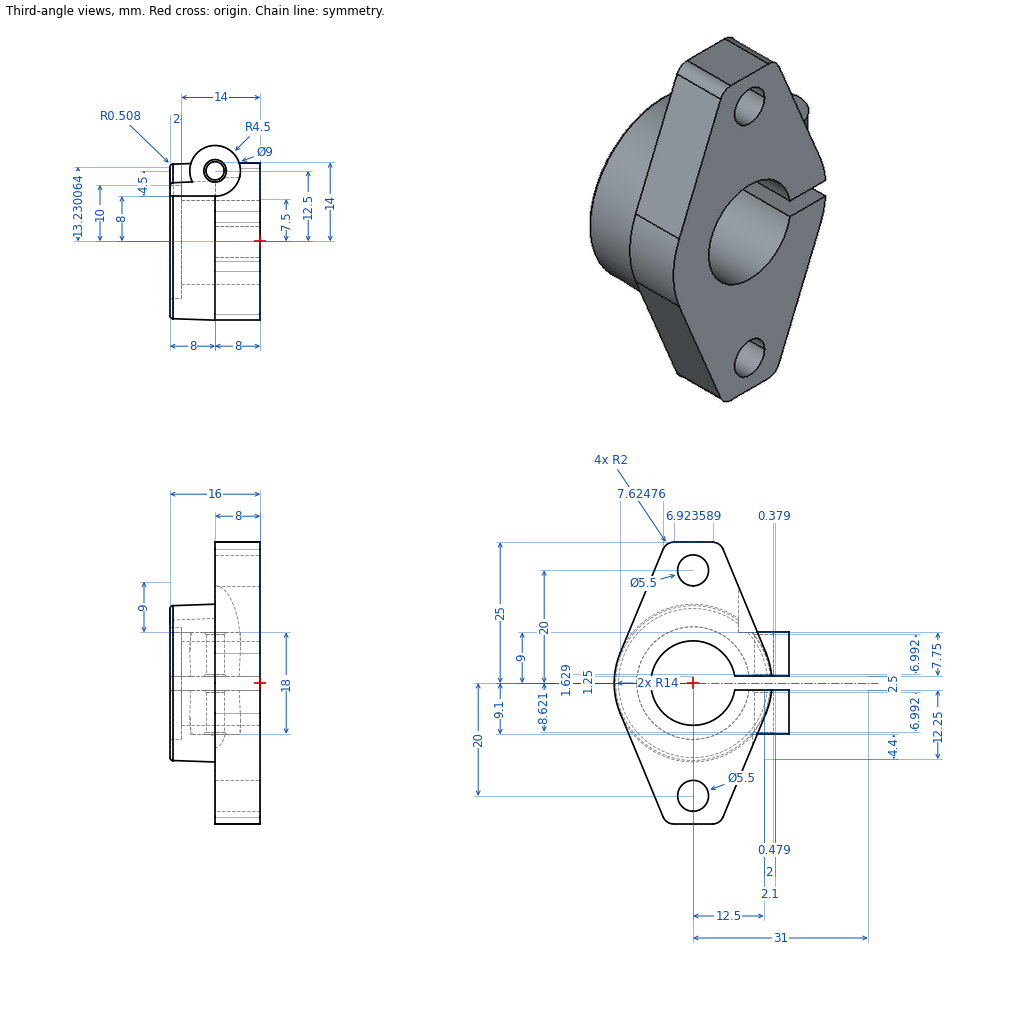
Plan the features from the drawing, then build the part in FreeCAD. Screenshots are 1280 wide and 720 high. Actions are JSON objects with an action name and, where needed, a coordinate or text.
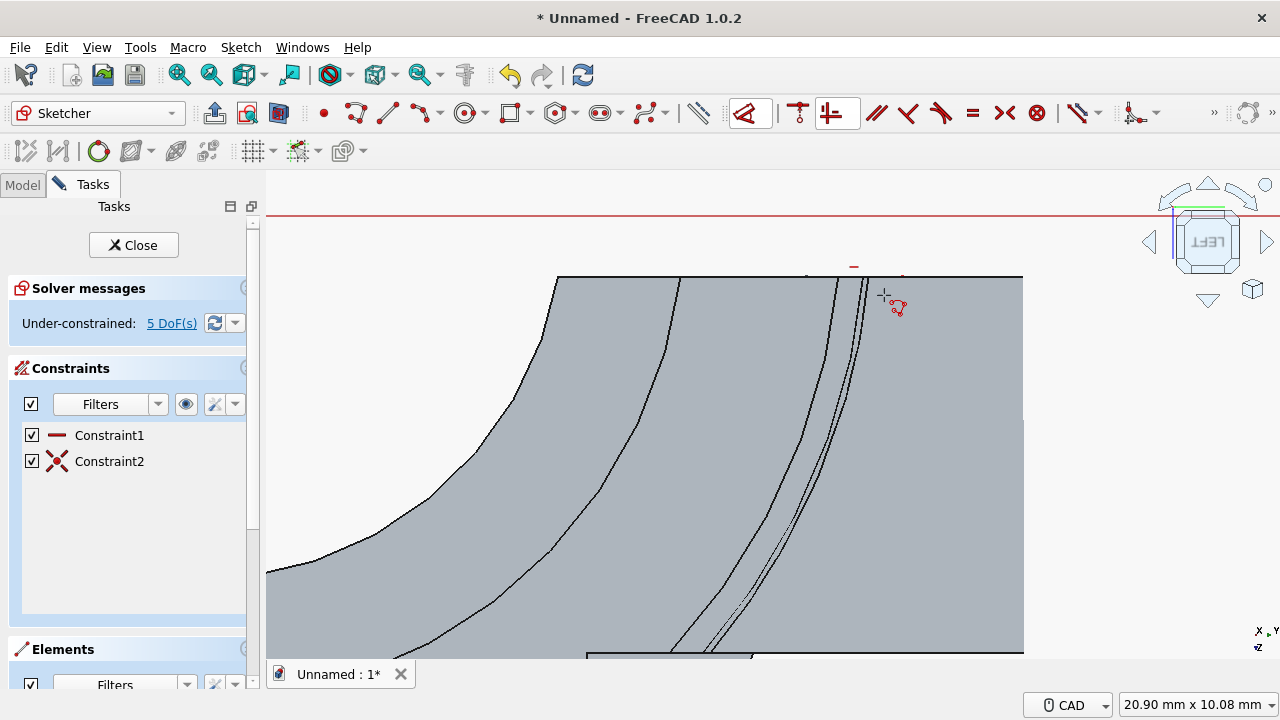
{"action": "scroll", "coordinate": [891, 299], "scroll_direction": "down", "scroll_amount": 3}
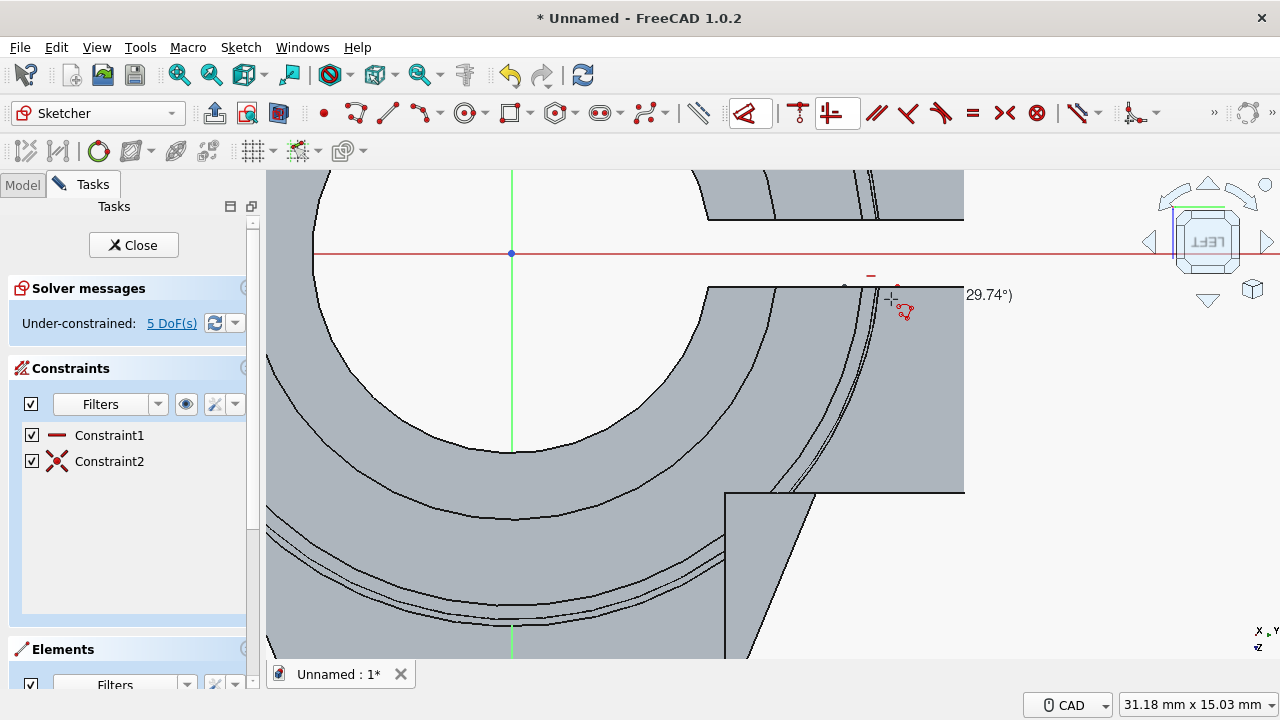
{"action": "left_click", "coordinate": [887, 483]}
{"action": "left_click", "coordinate": [898, 493]}
{"action": "left_click", "coordinate": [845, 493]}
{"action": "left_click", "coordinate": [845, 288]}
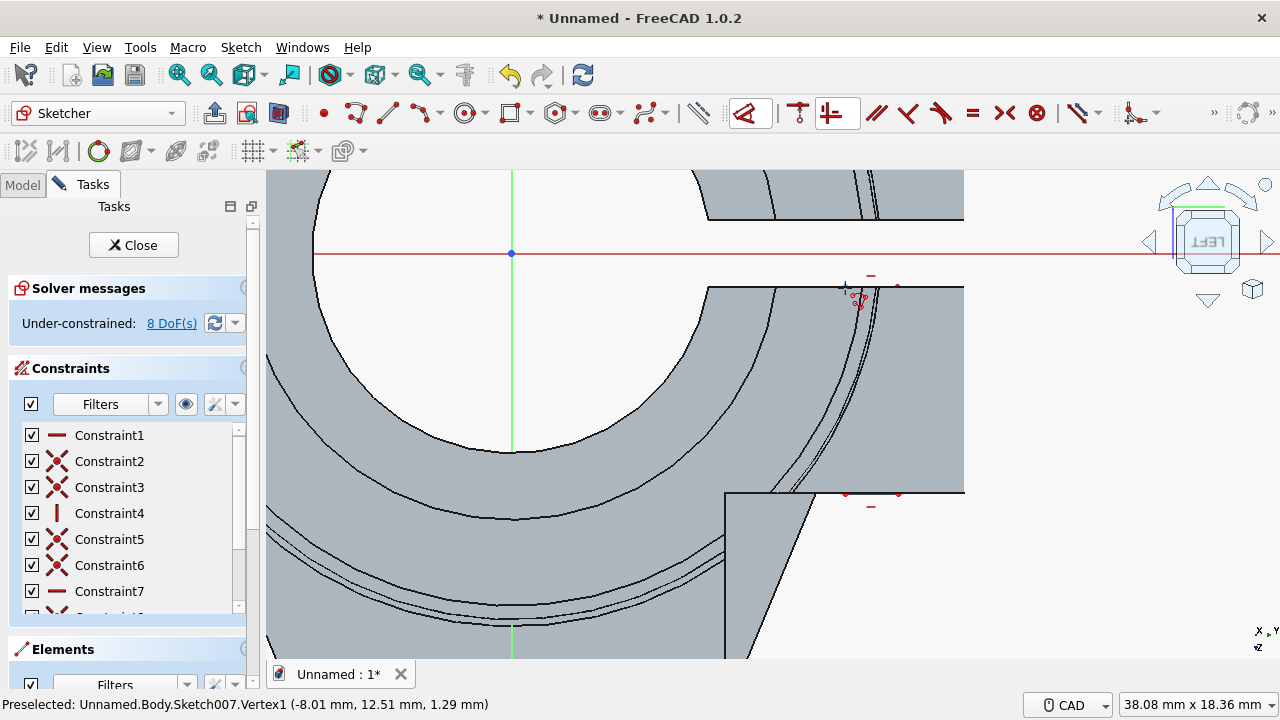
{"action": "left_click", "coordinate": [388, 114]}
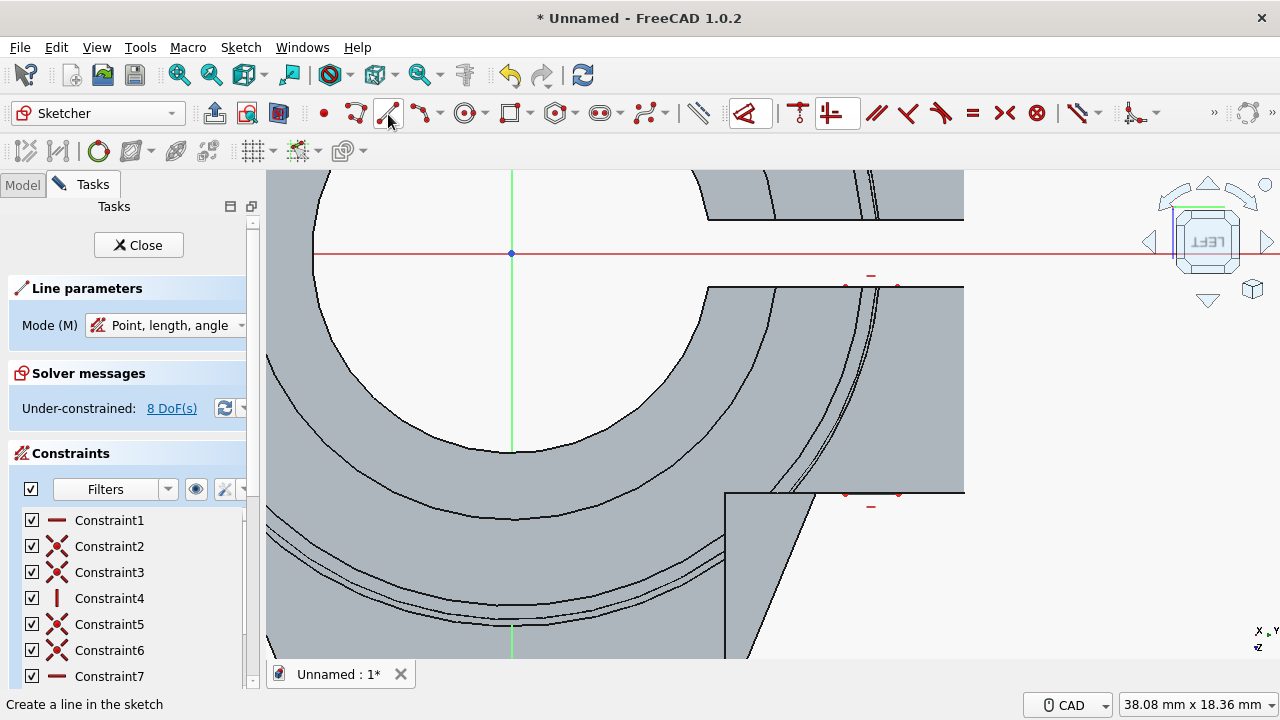
{"action": "left_click", "coordinate": [845, 514]}
{"action": "left_click", "coordinate": [845, 576]}
{"action": "key", "text": "Escape"}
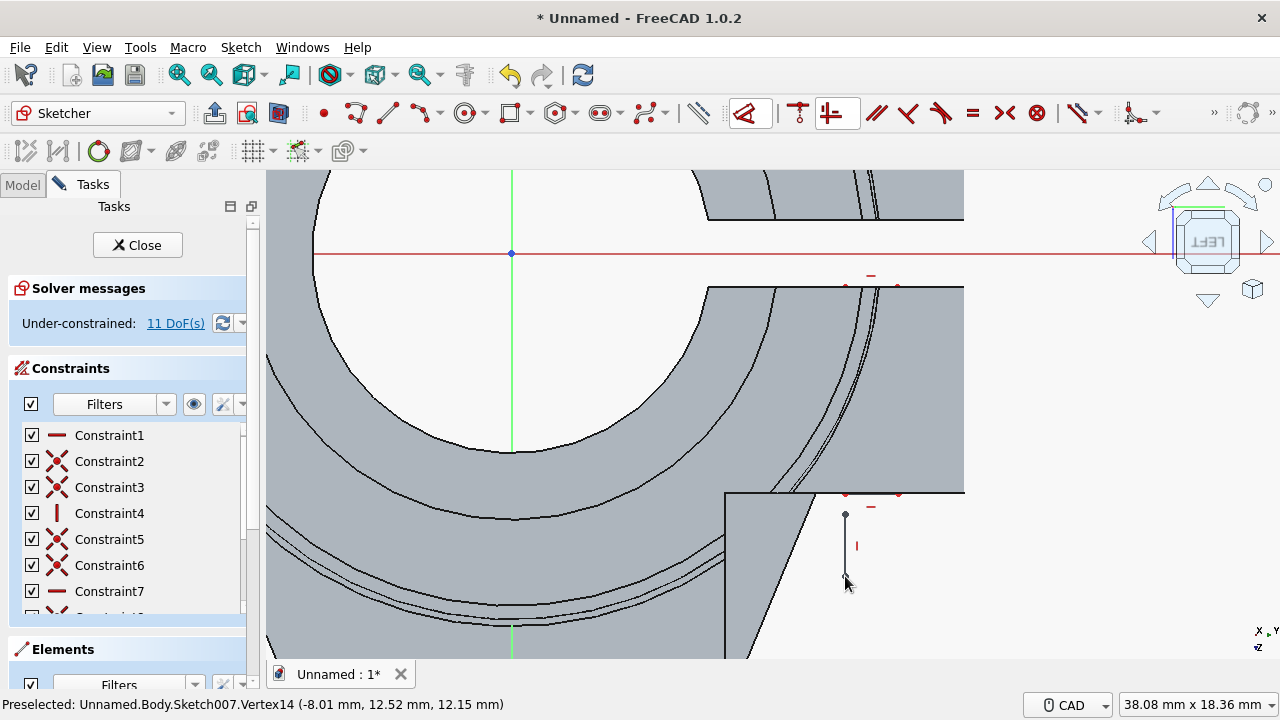
{"action": "left_click", "coordinate": [845, 534]}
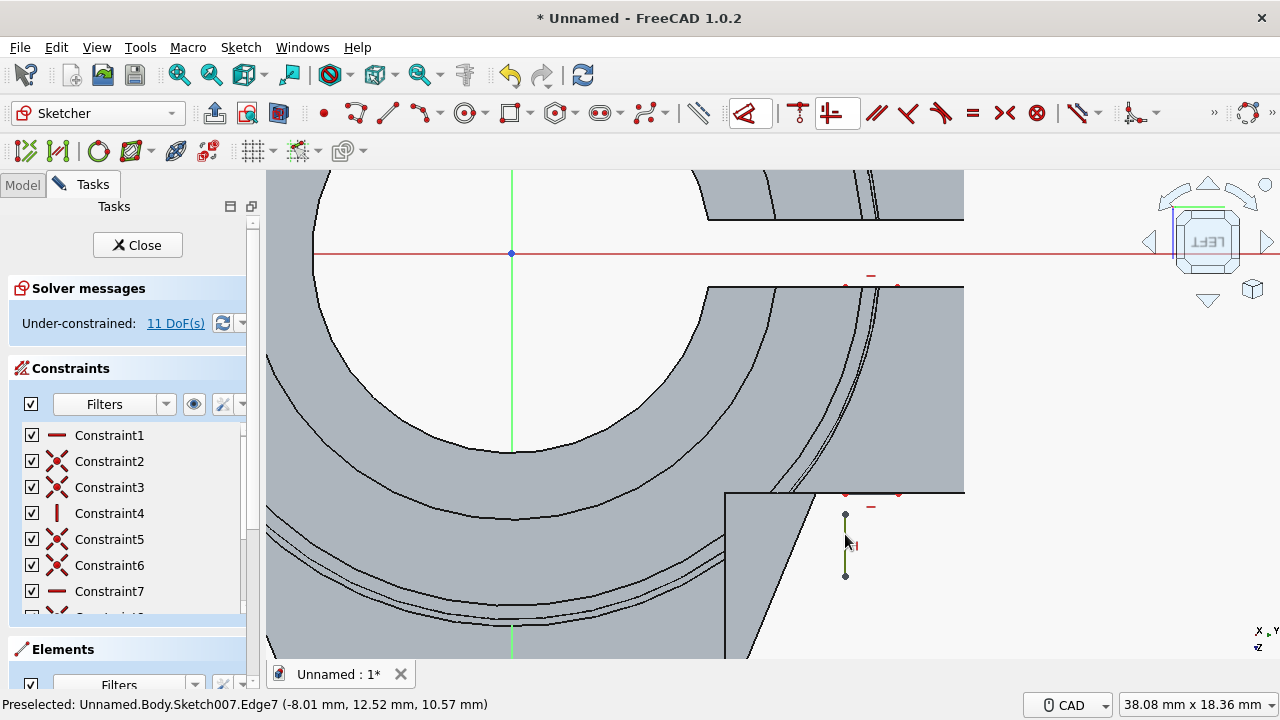
{"action": "left_click", "coordinate": [700, 114]}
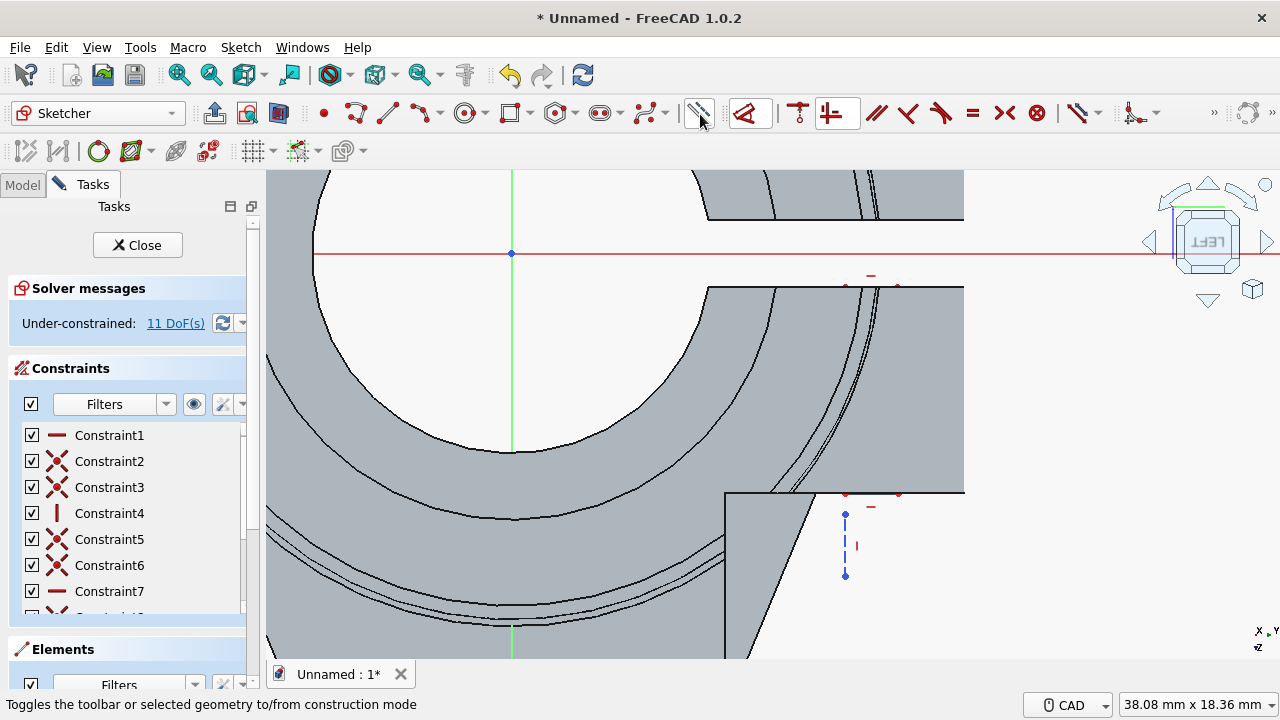
{"action": "left_click", "coordinate": [861, 288]}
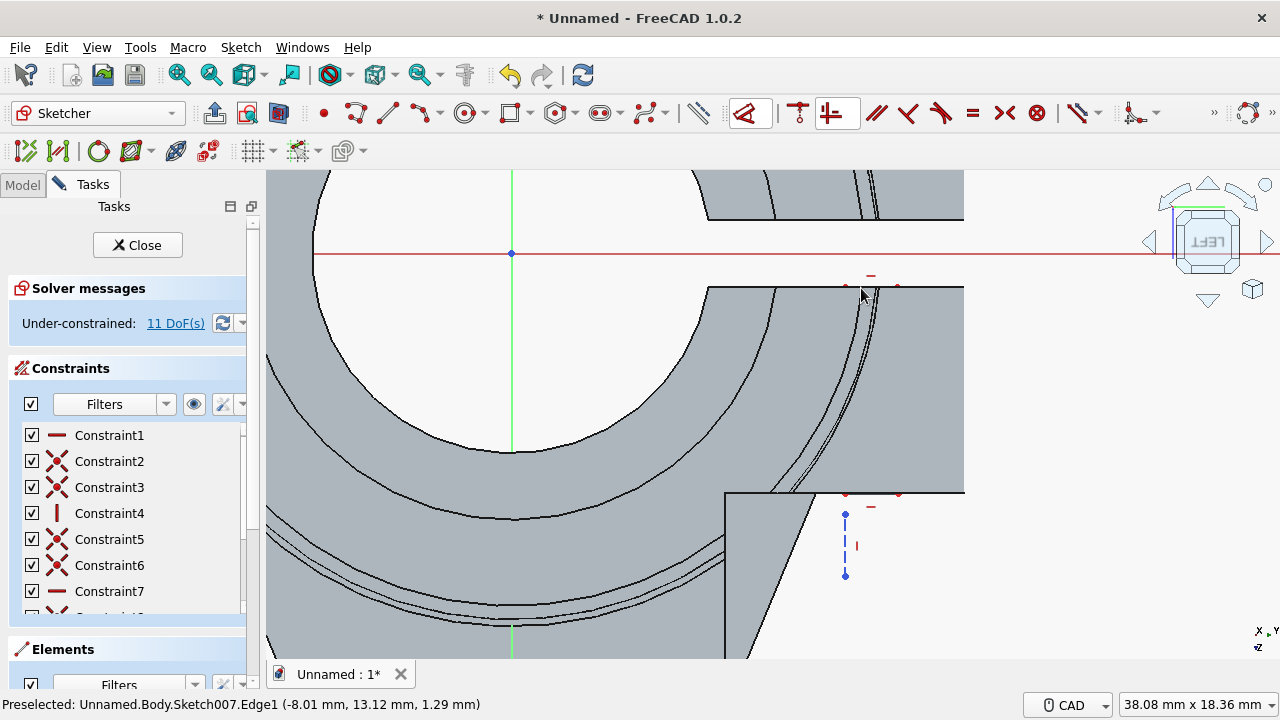
{"action": "left_click", "coordinate": [766, 114]}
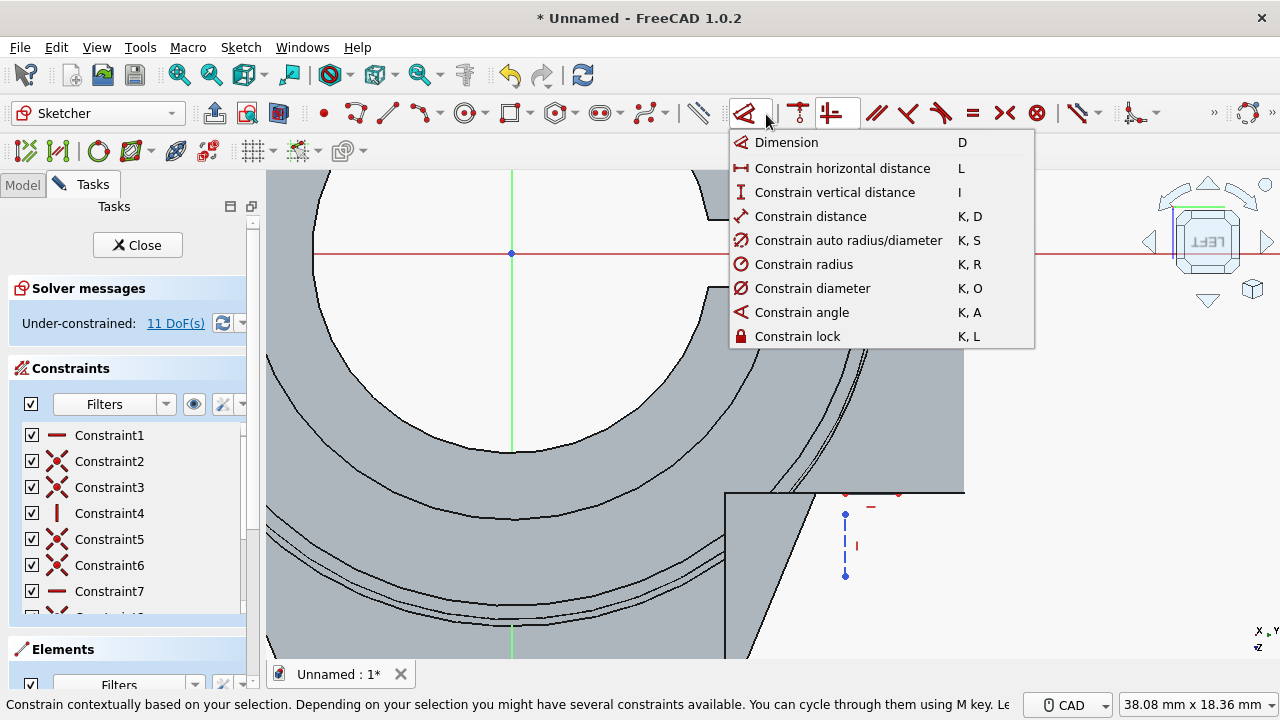
{"action": "left_click", "coordinate": [882, 168]}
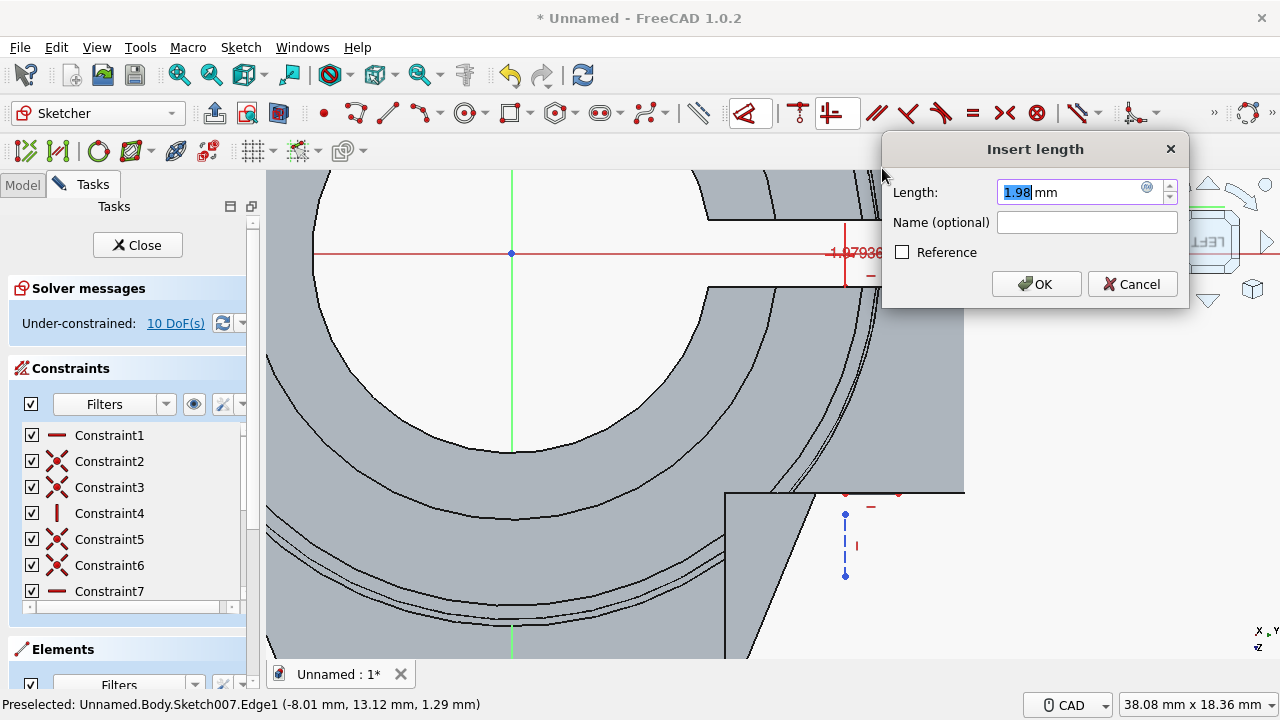
{"action": "type", "text": "2"}
{"action": "key", "text": "Return"}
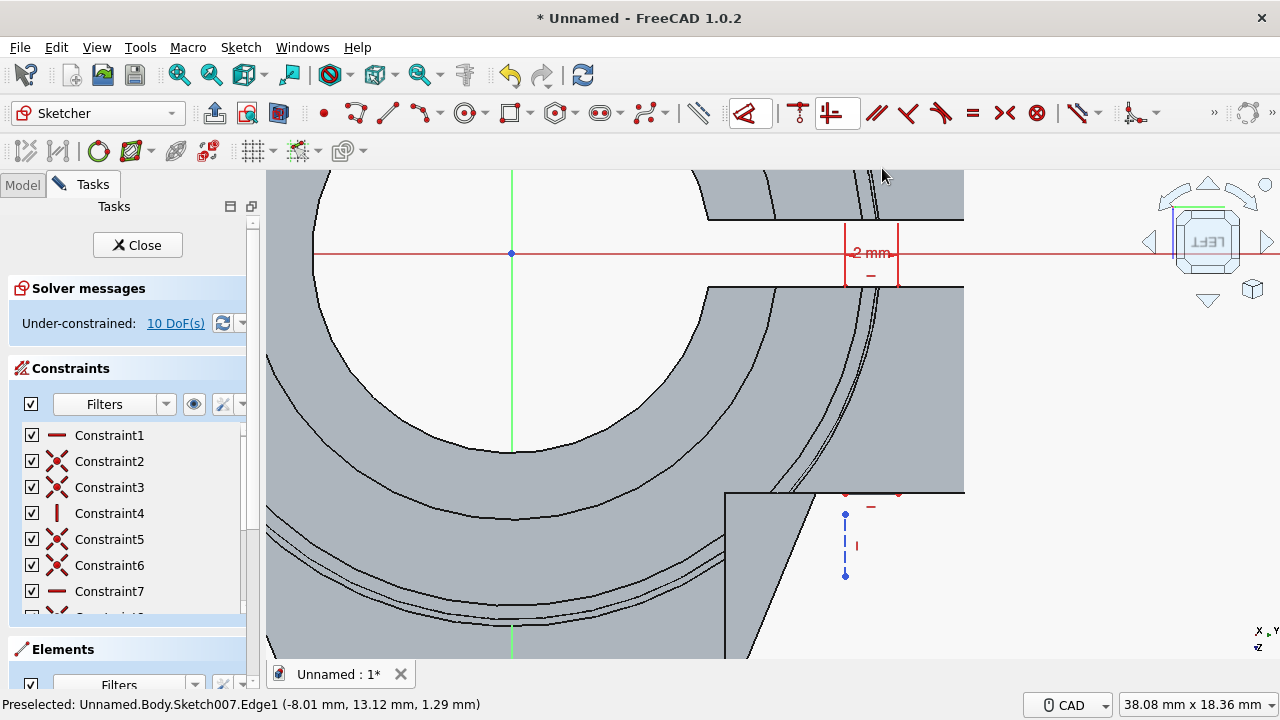
{"action": "scroll", "coordinate": [882, 494], "scroll_direction": "up", "scroll_amount": 2}